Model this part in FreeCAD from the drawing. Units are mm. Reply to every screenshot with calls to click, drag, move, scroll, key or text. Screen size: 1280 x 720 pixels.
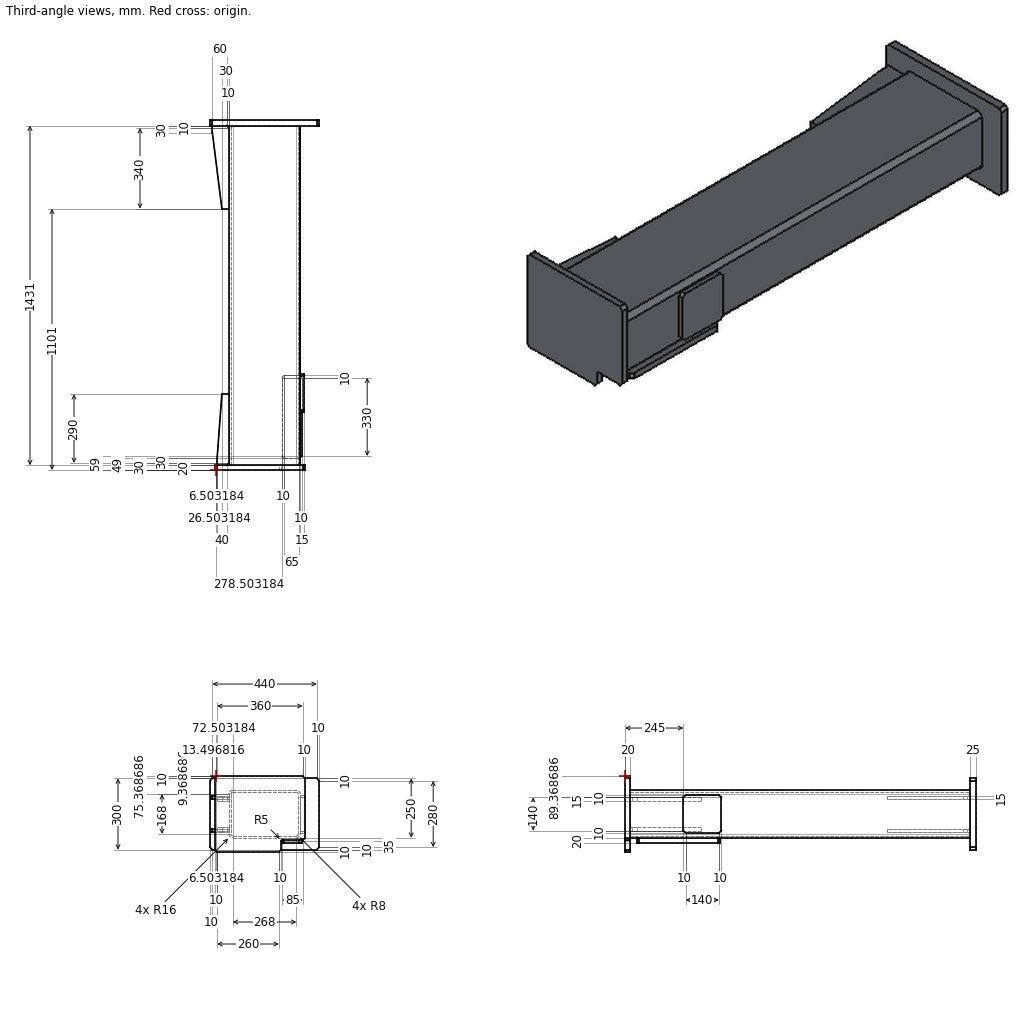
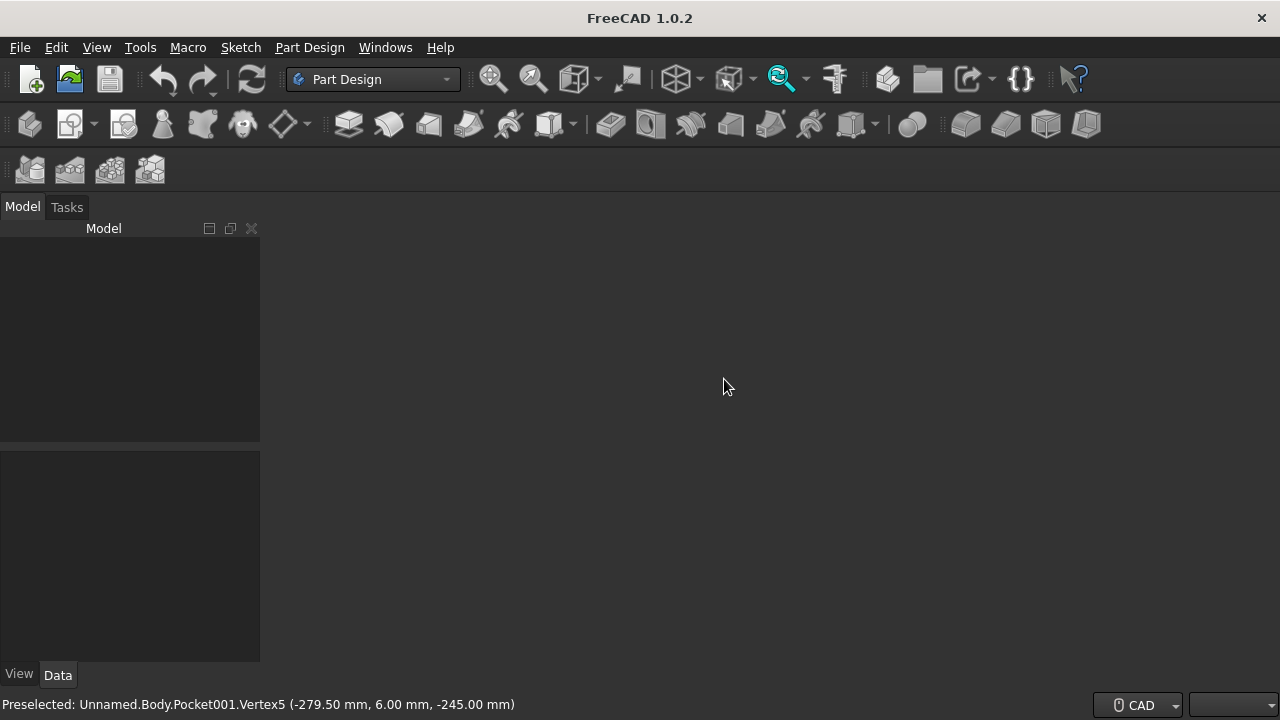
click(30, 80)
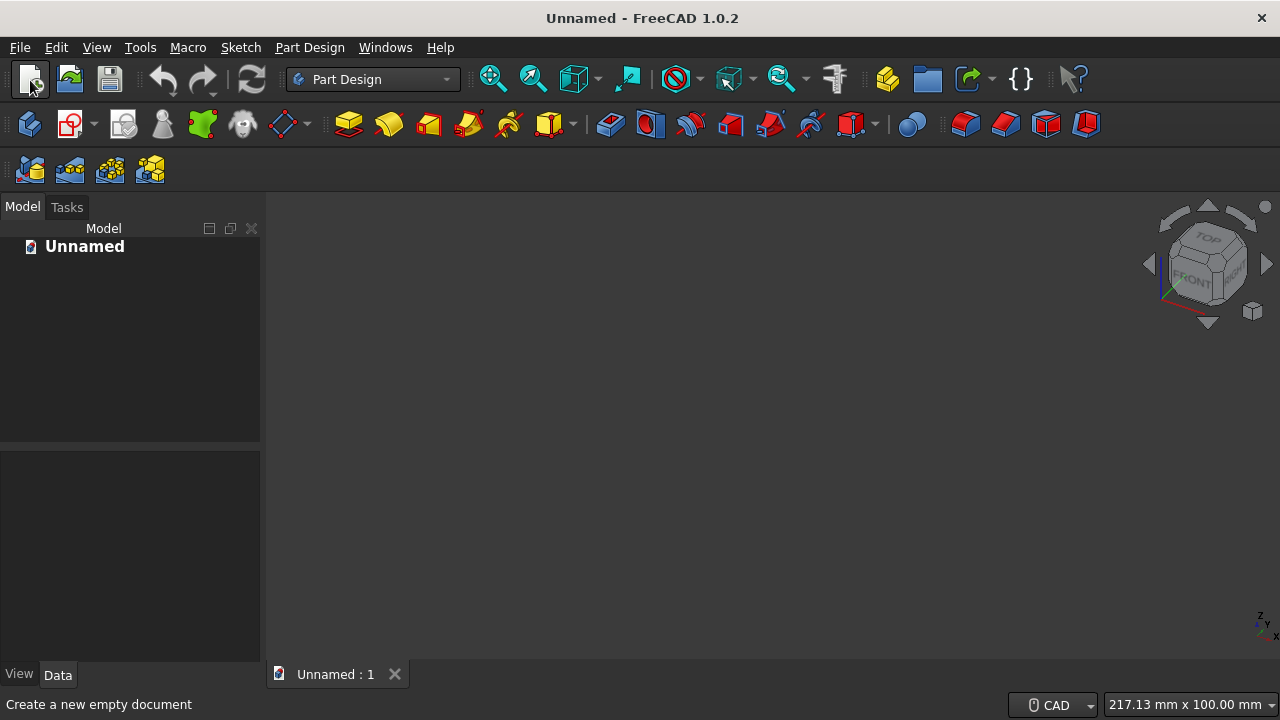
click(70, 124)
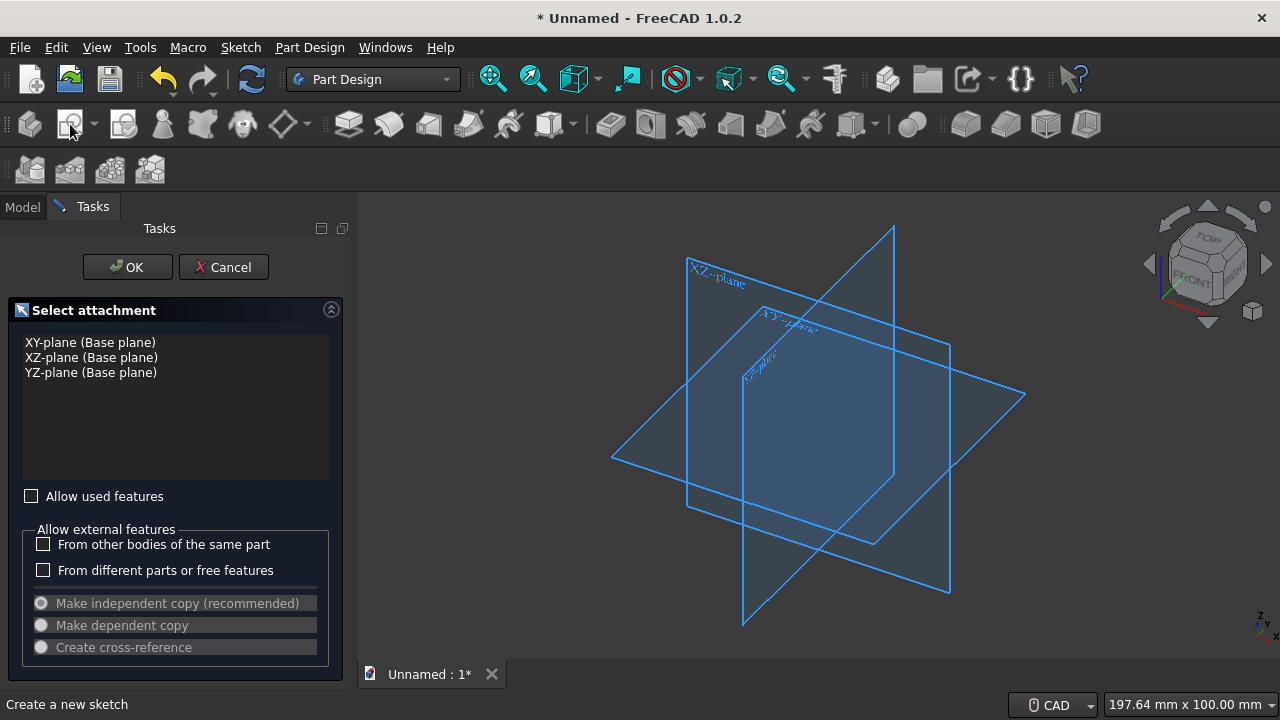
click(82, 358)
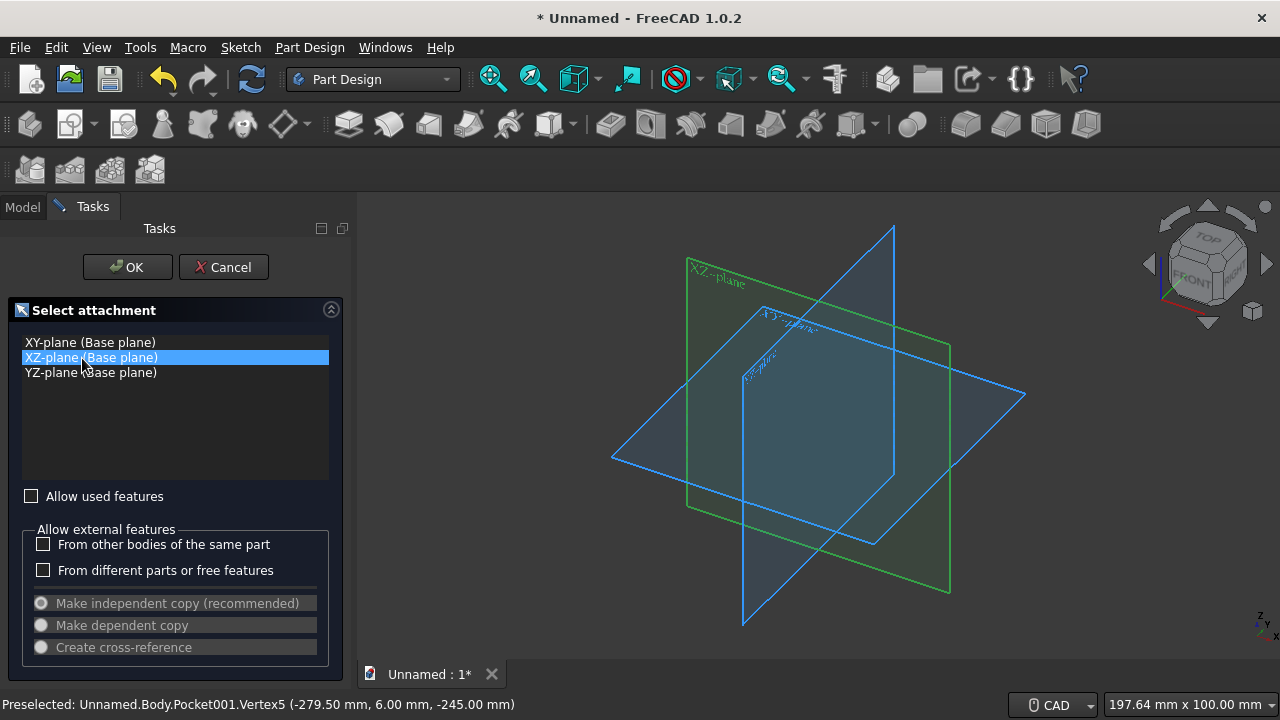
click(128, 267)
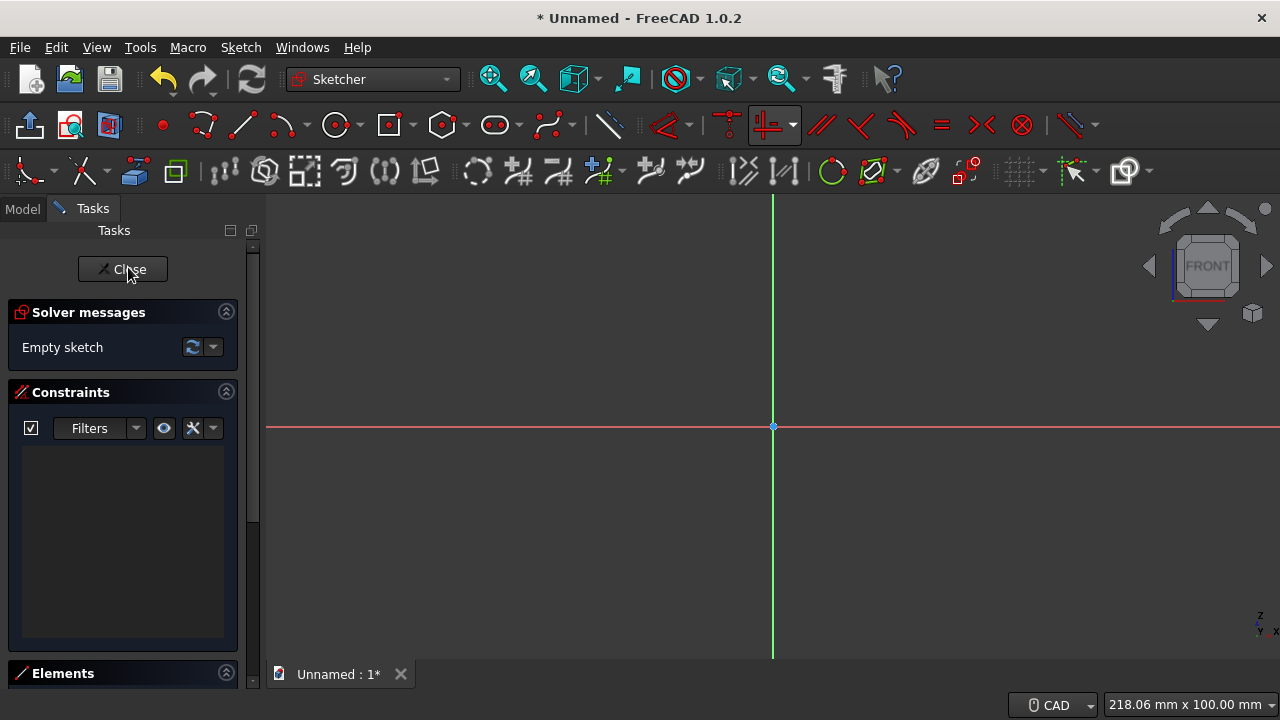
scroll(468, 239, down, 8)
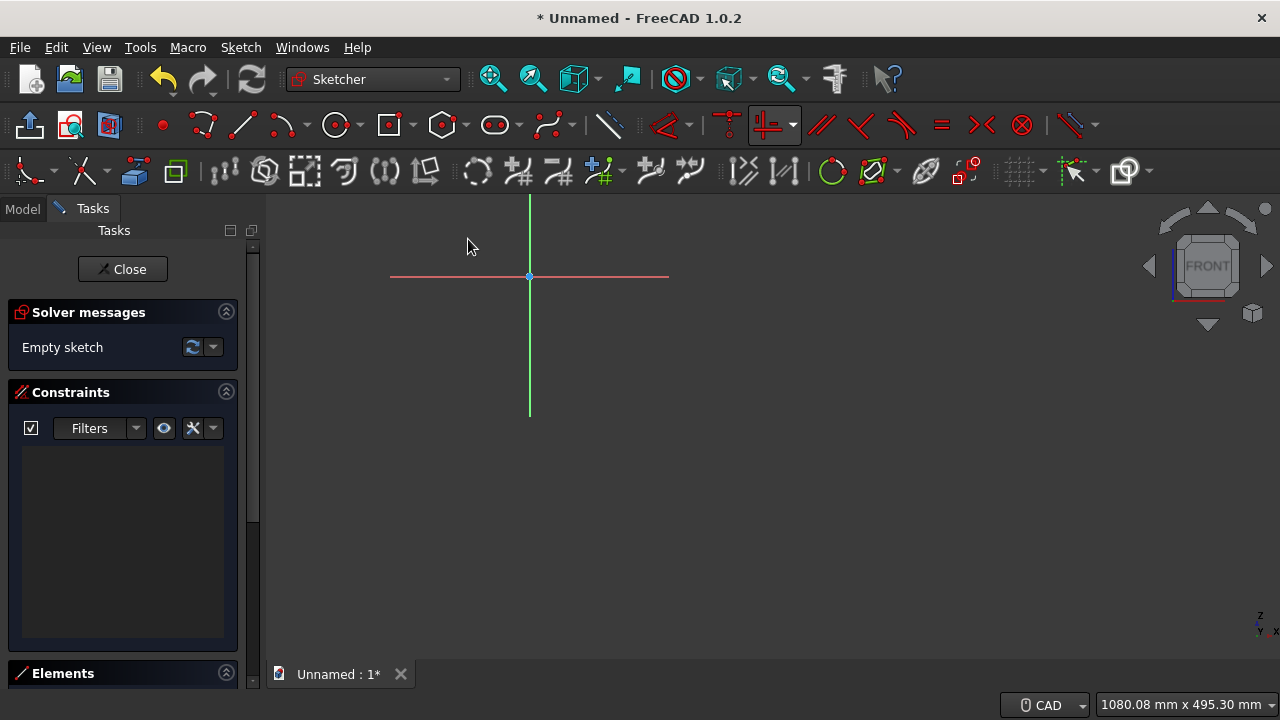
key(g)
key(m)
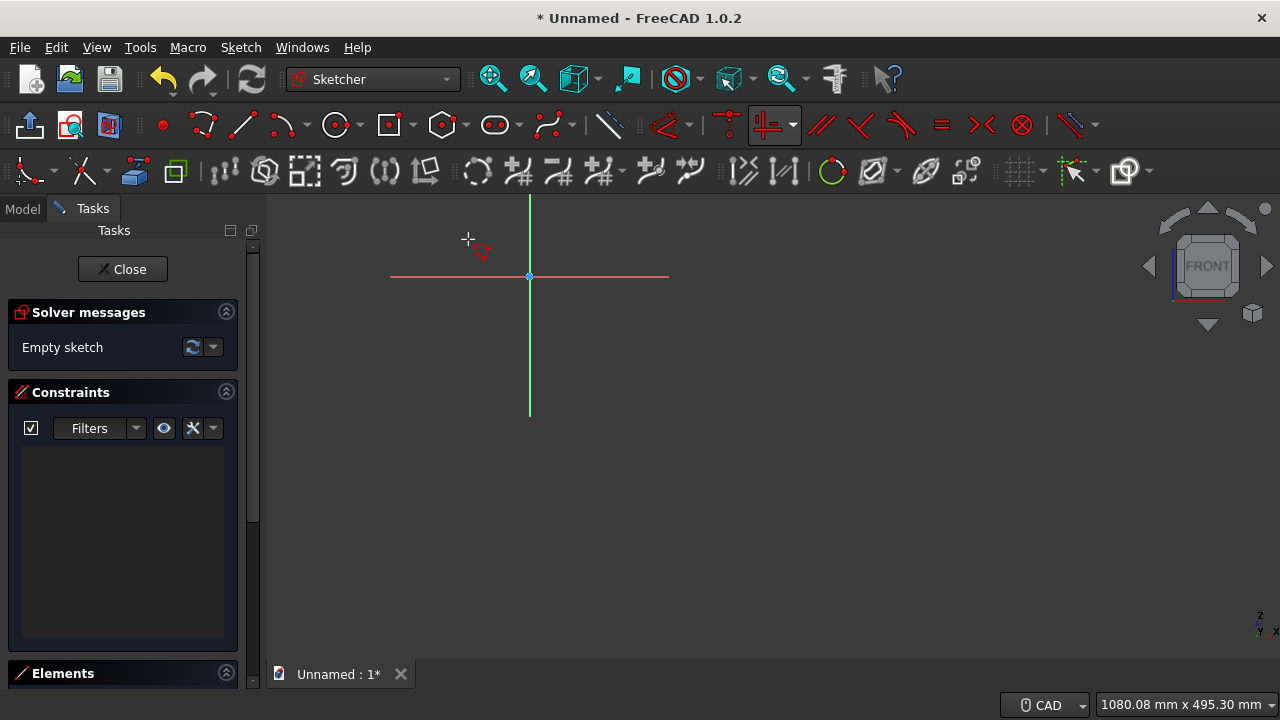
click(789, 535)
click(789, 567)
click(780, 577)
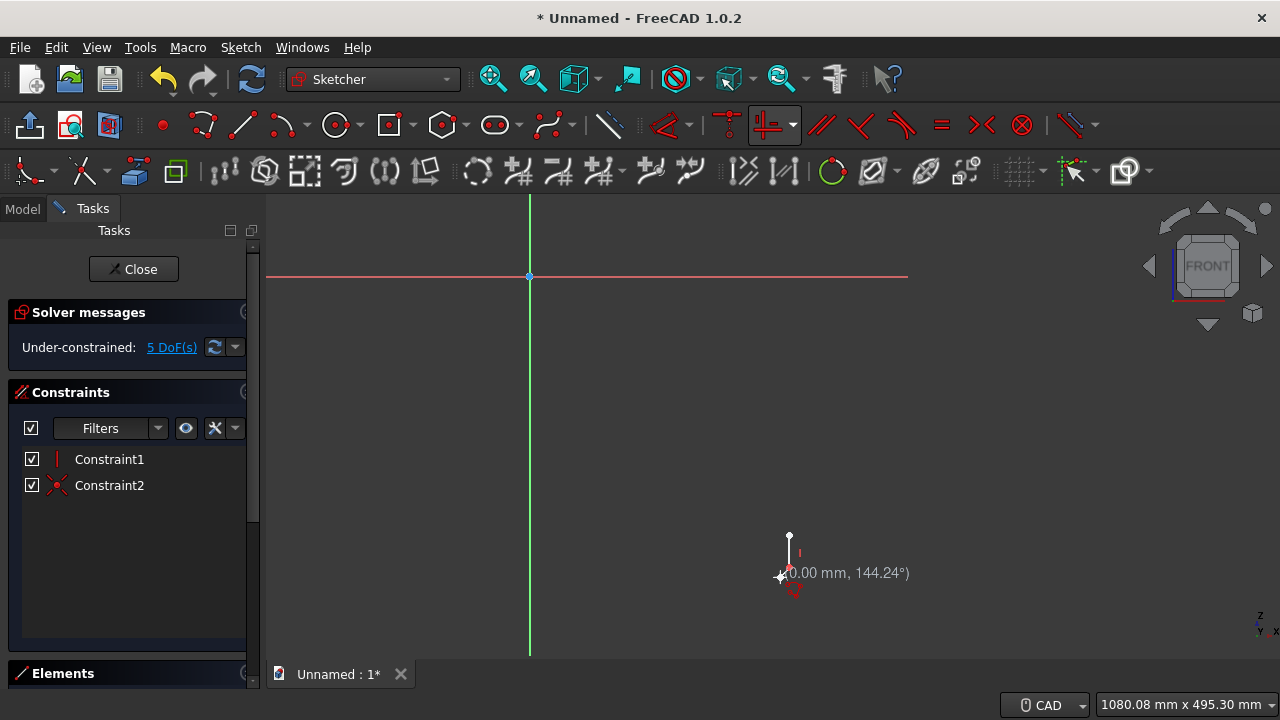
scroll(536, 577, up, 5)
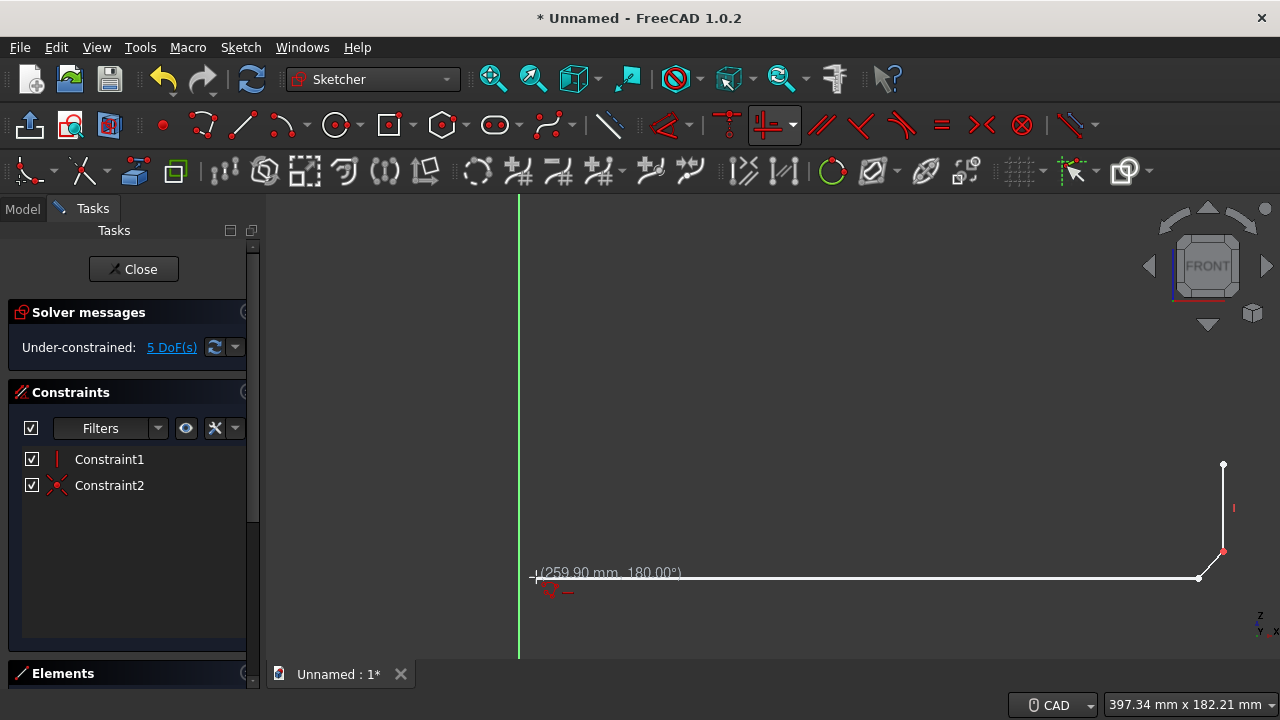
click(535, 576)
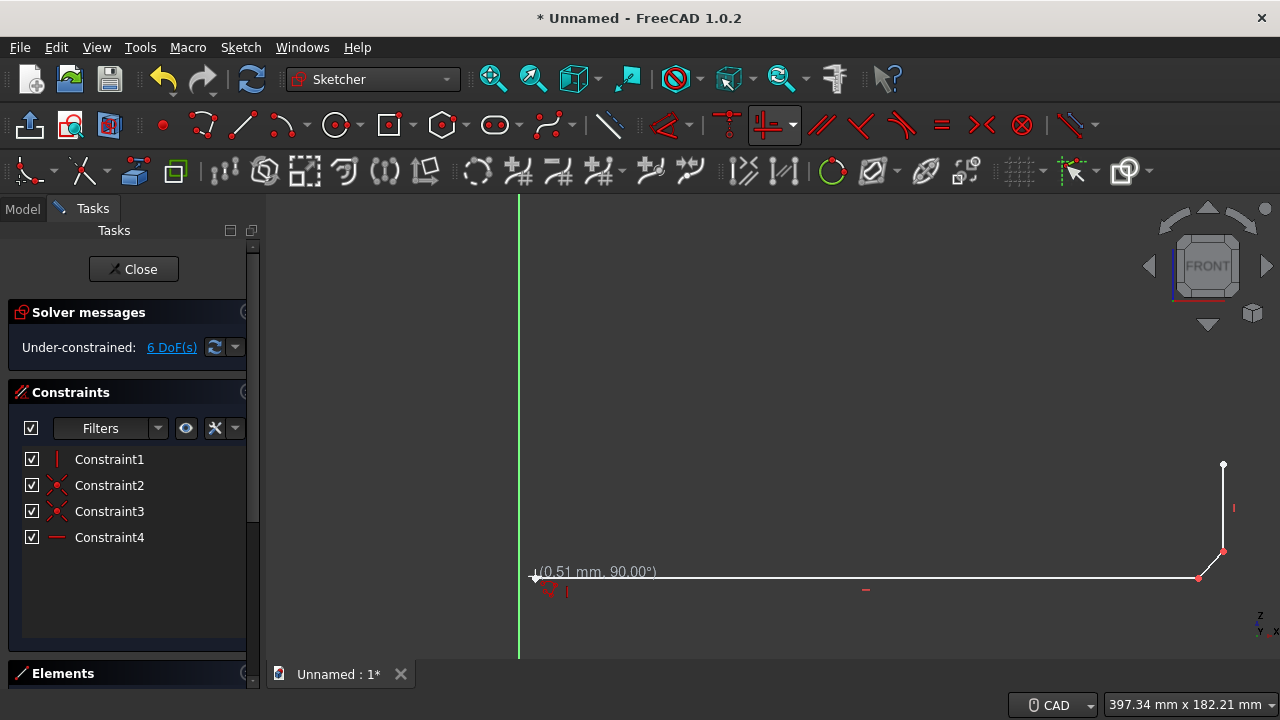
scroll(510, 549, up, 3)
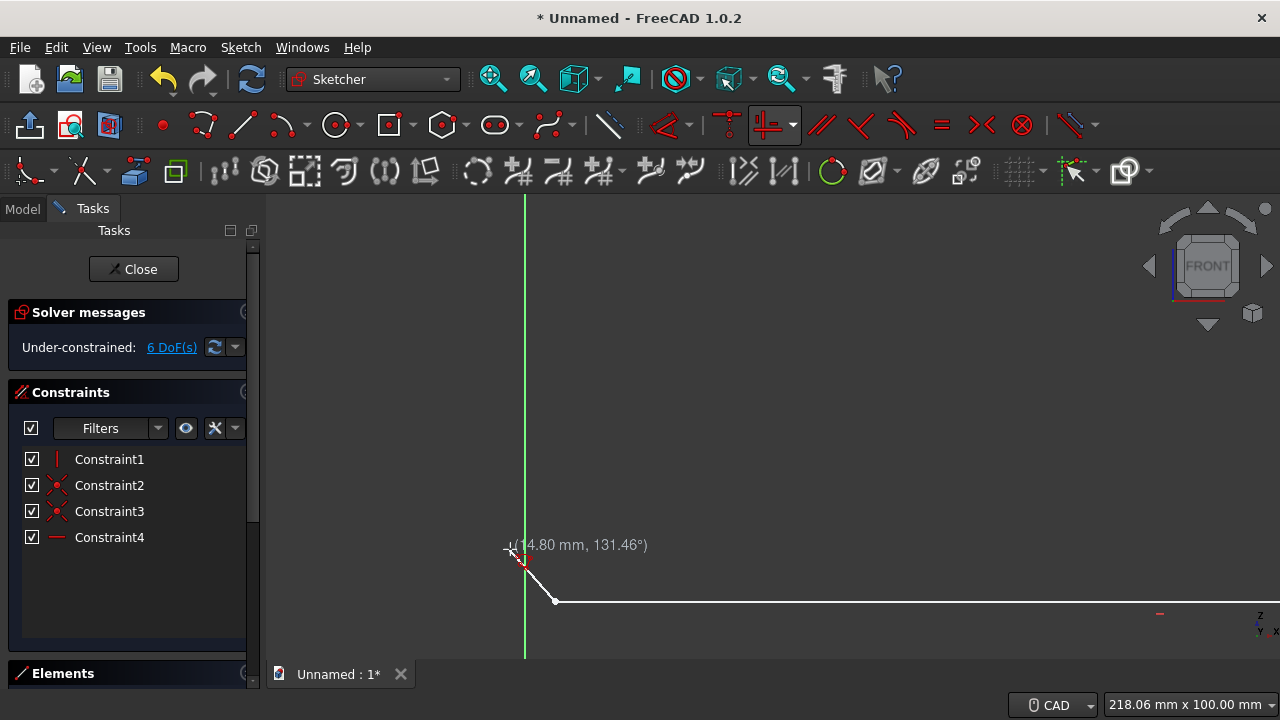
click(509, 549)